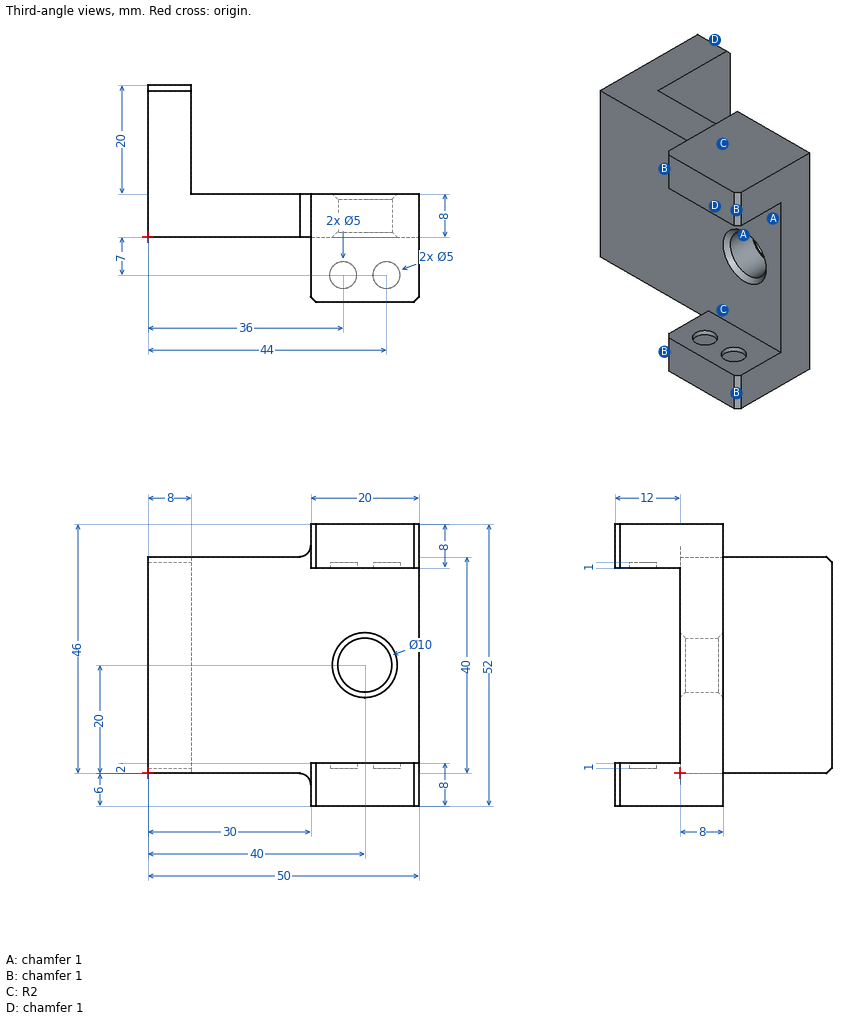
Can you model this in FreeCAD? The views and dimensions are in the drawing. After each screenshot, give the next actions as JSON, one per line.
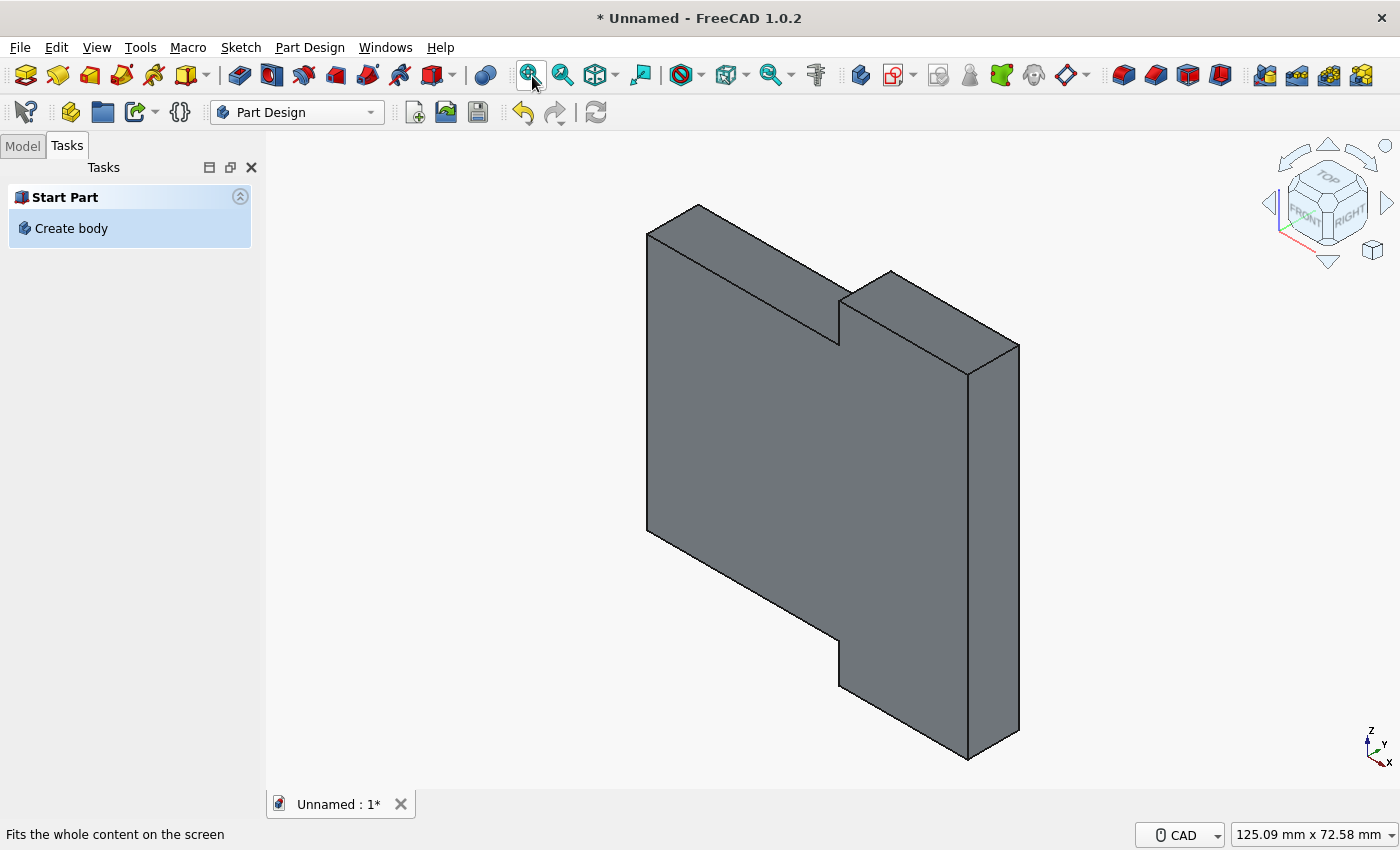
{"action": "left_click", "coordinate": [807, 474]}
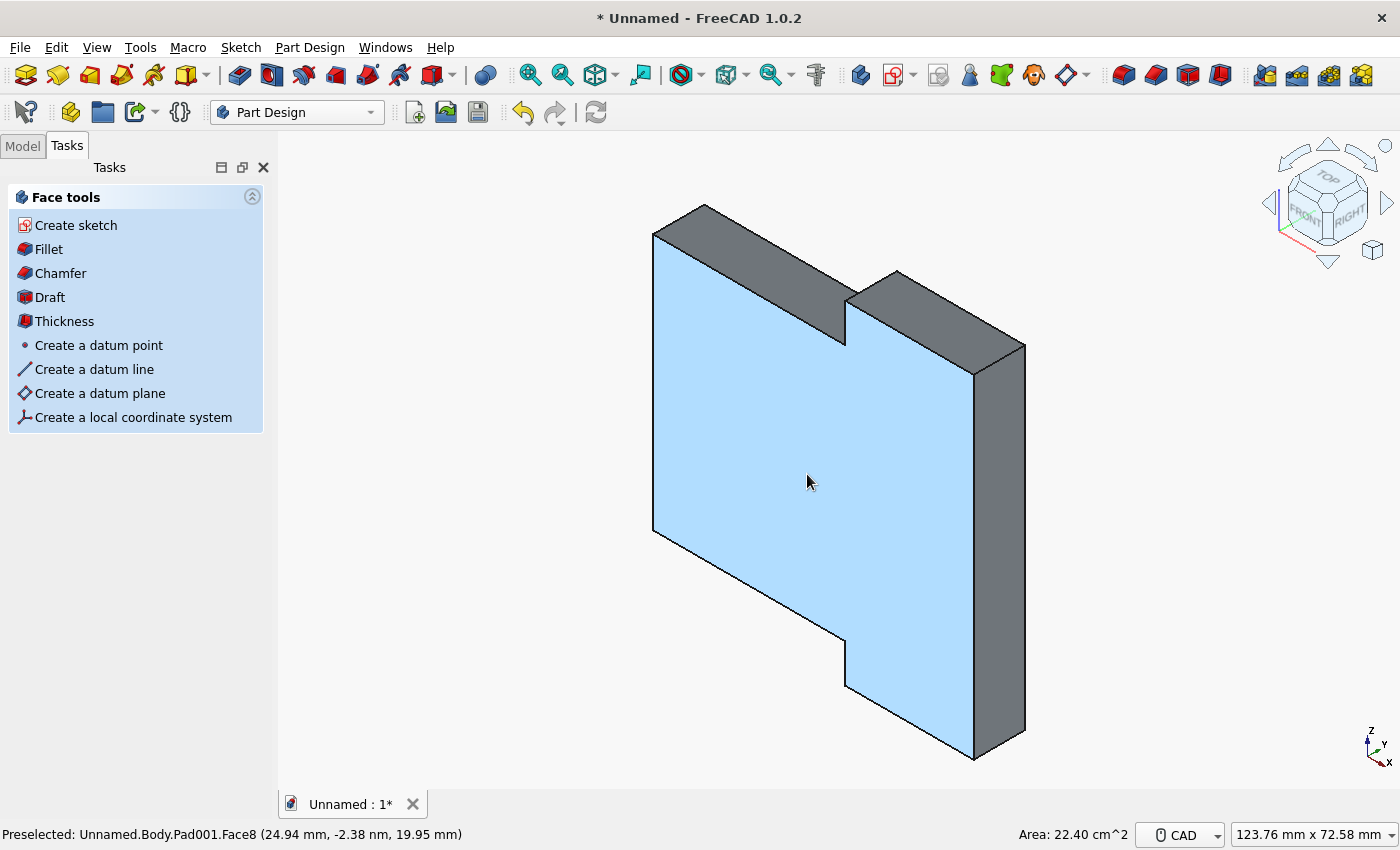
{"action": "left_click", "coordinate": [894, 76]}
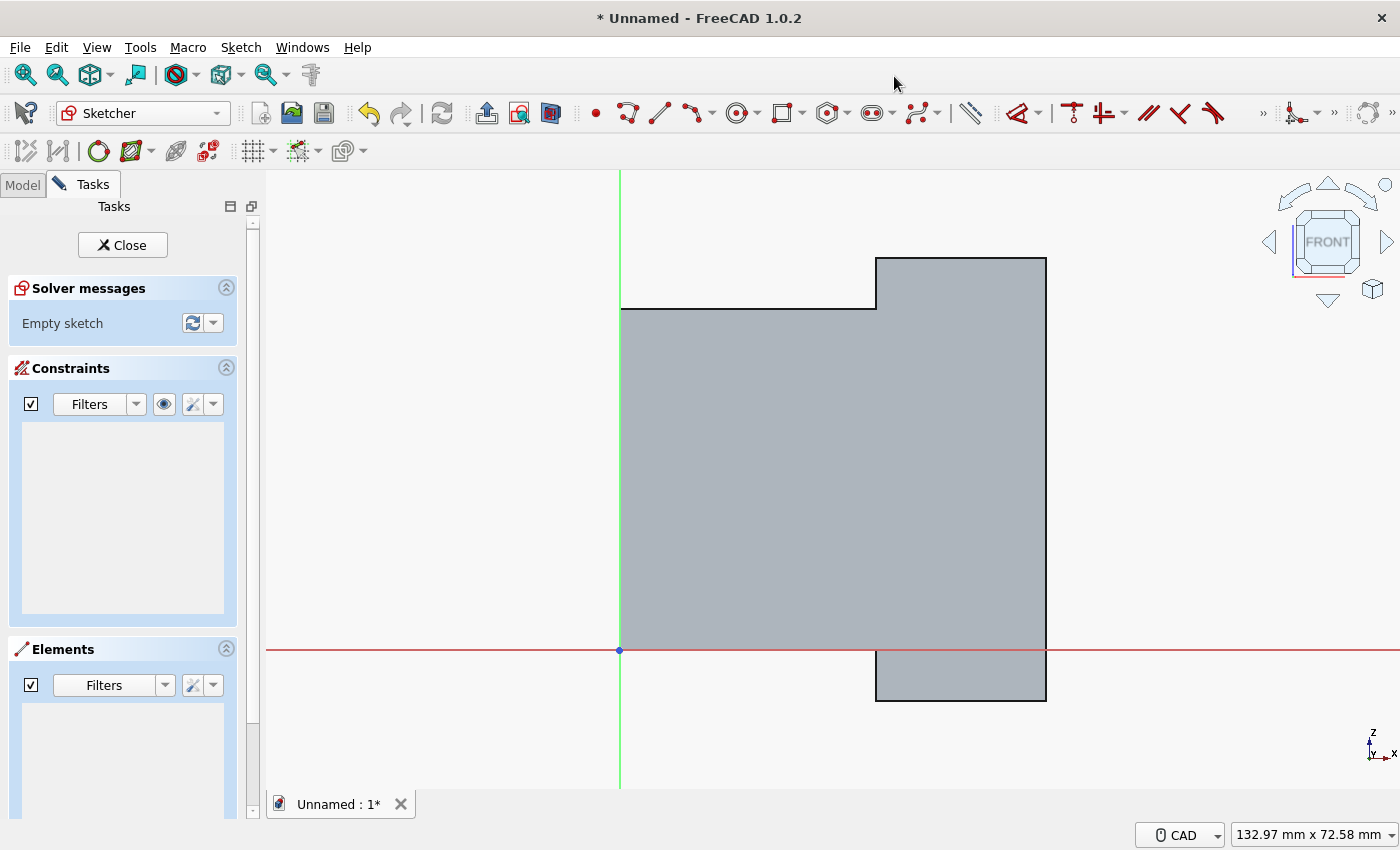
{"action": "scroll", "coordinate": [1011, 480], "scroll_direction": "up", "scroll_amount": 8}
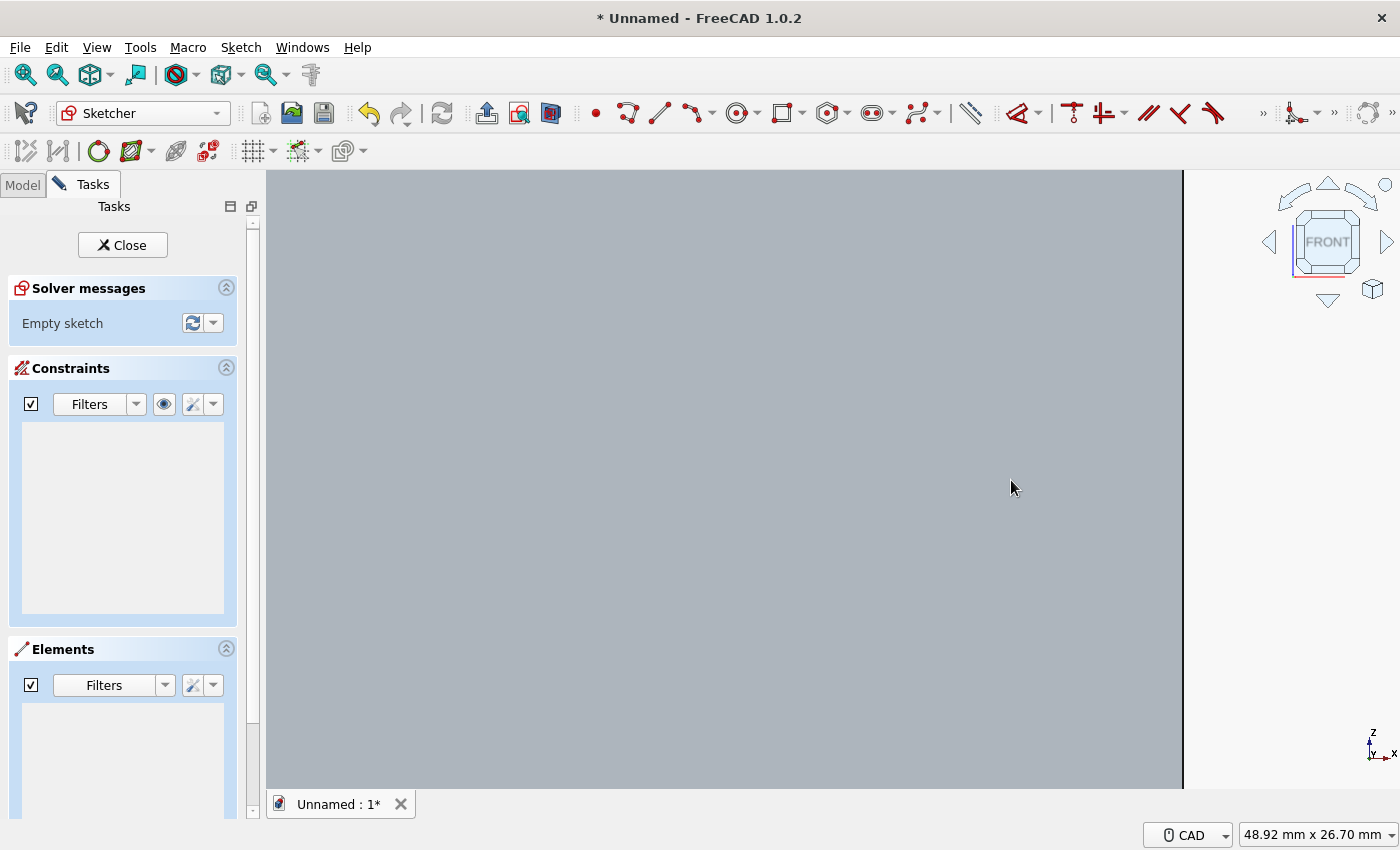
{"action": "left_click", "coordinate": [738, 114]}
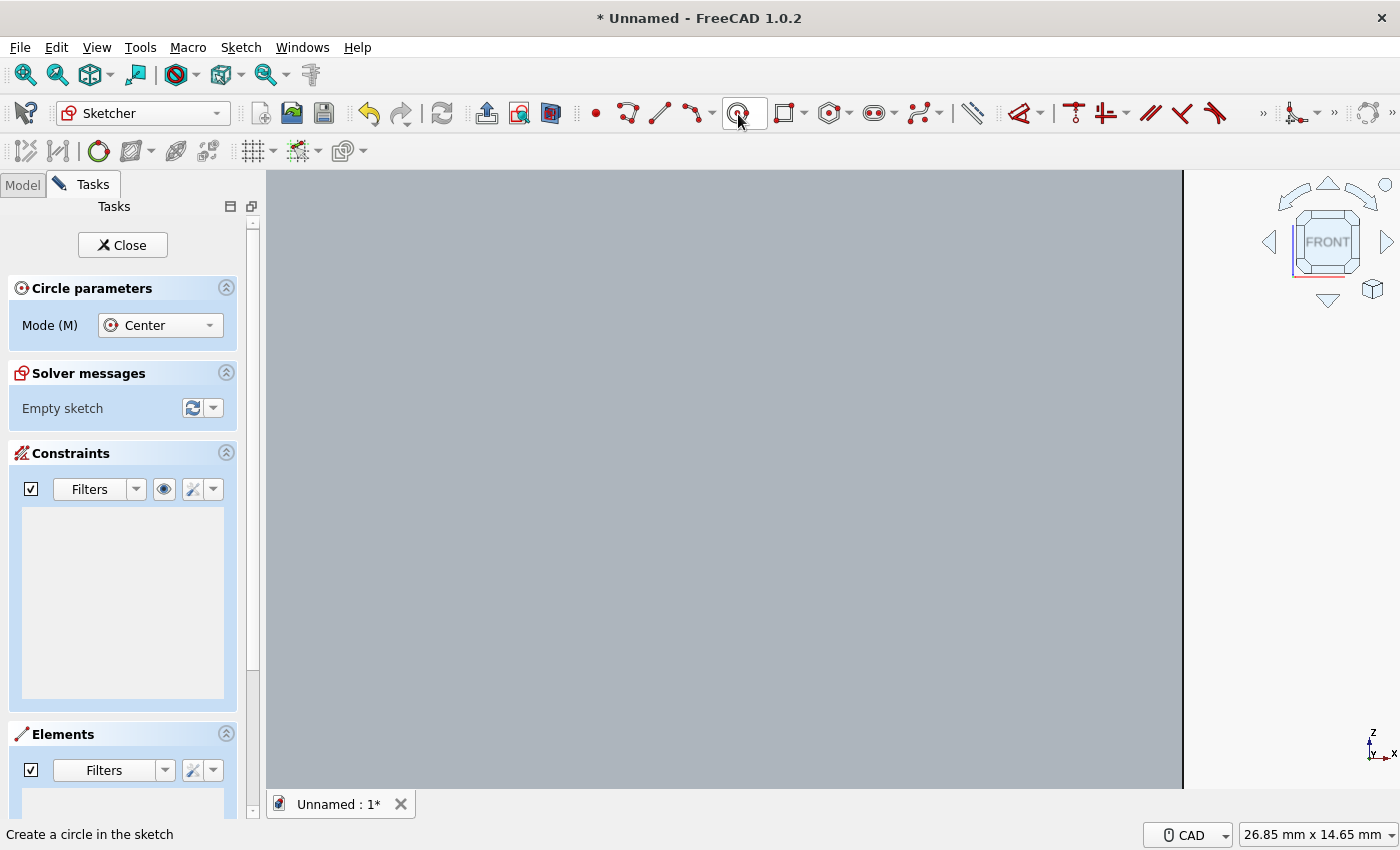
{"action": "left_click", "coordinate": [760, 476]}
{"action": "mouse_move", "coordinate": [910, 326]}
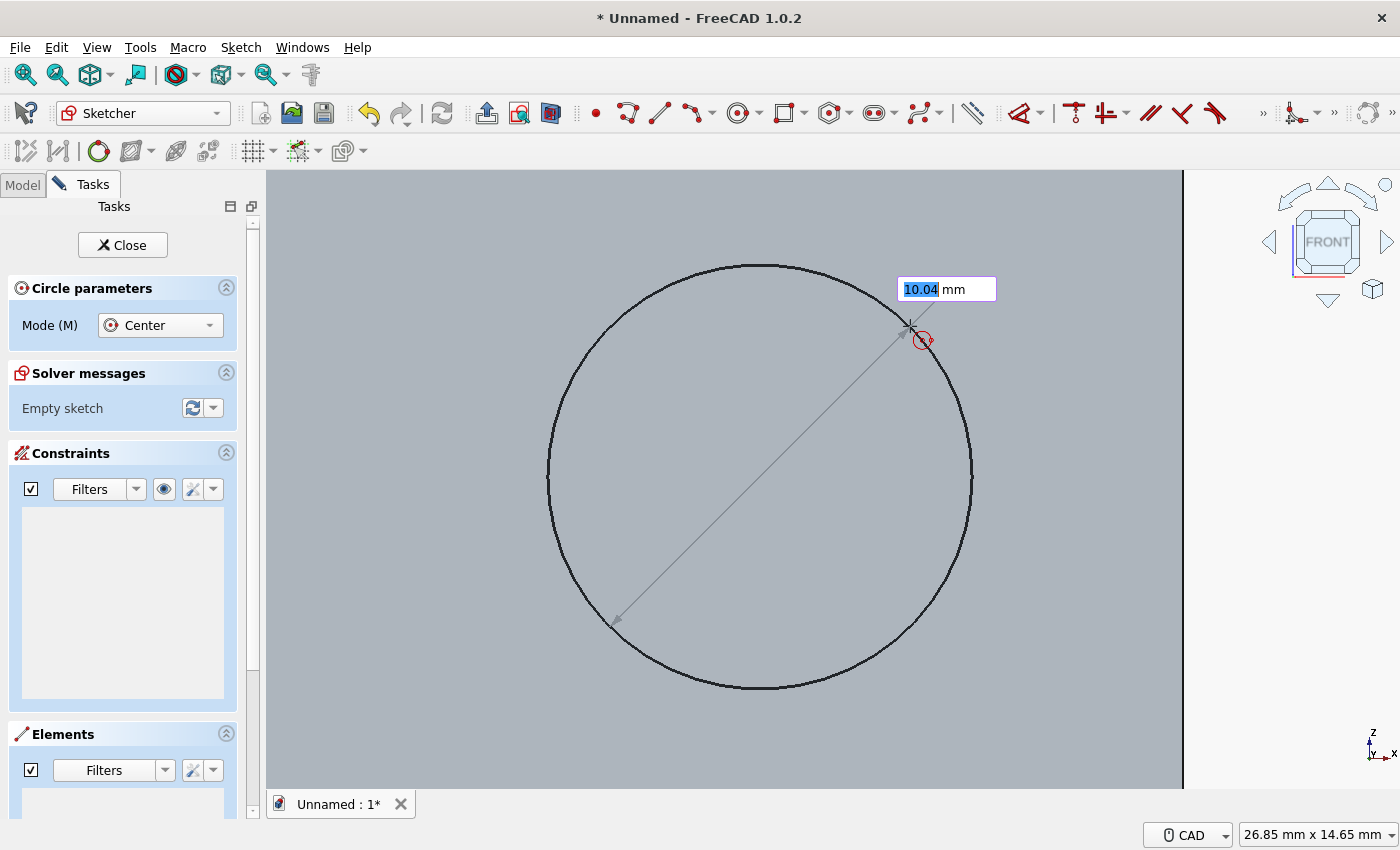
{"action": "type", "text": "10"}
{"action": "key", "text": "Return"}
{"action": "key", "text": "Escape"}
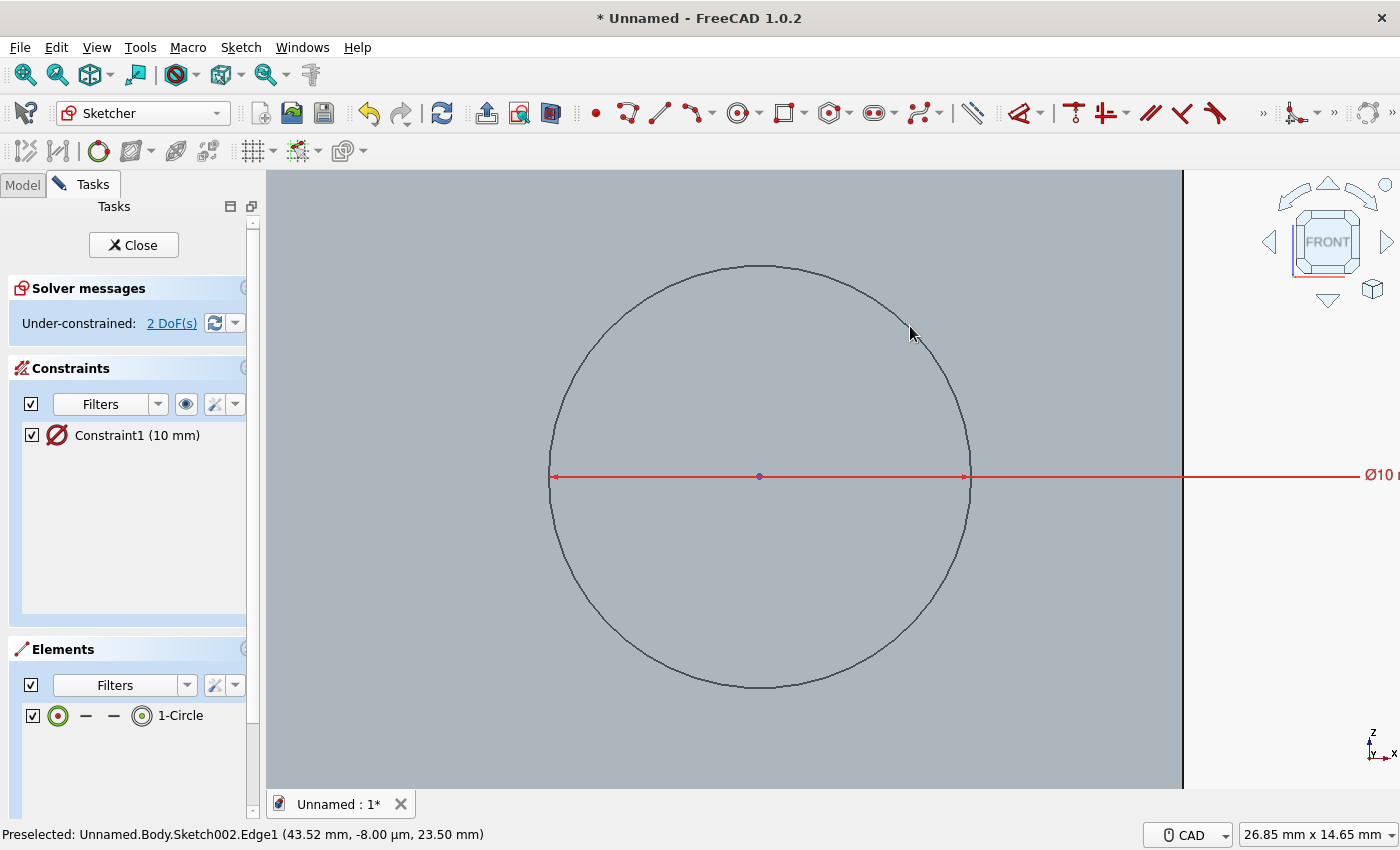
{"action": "left_click", "coordinate": [1020, 114]}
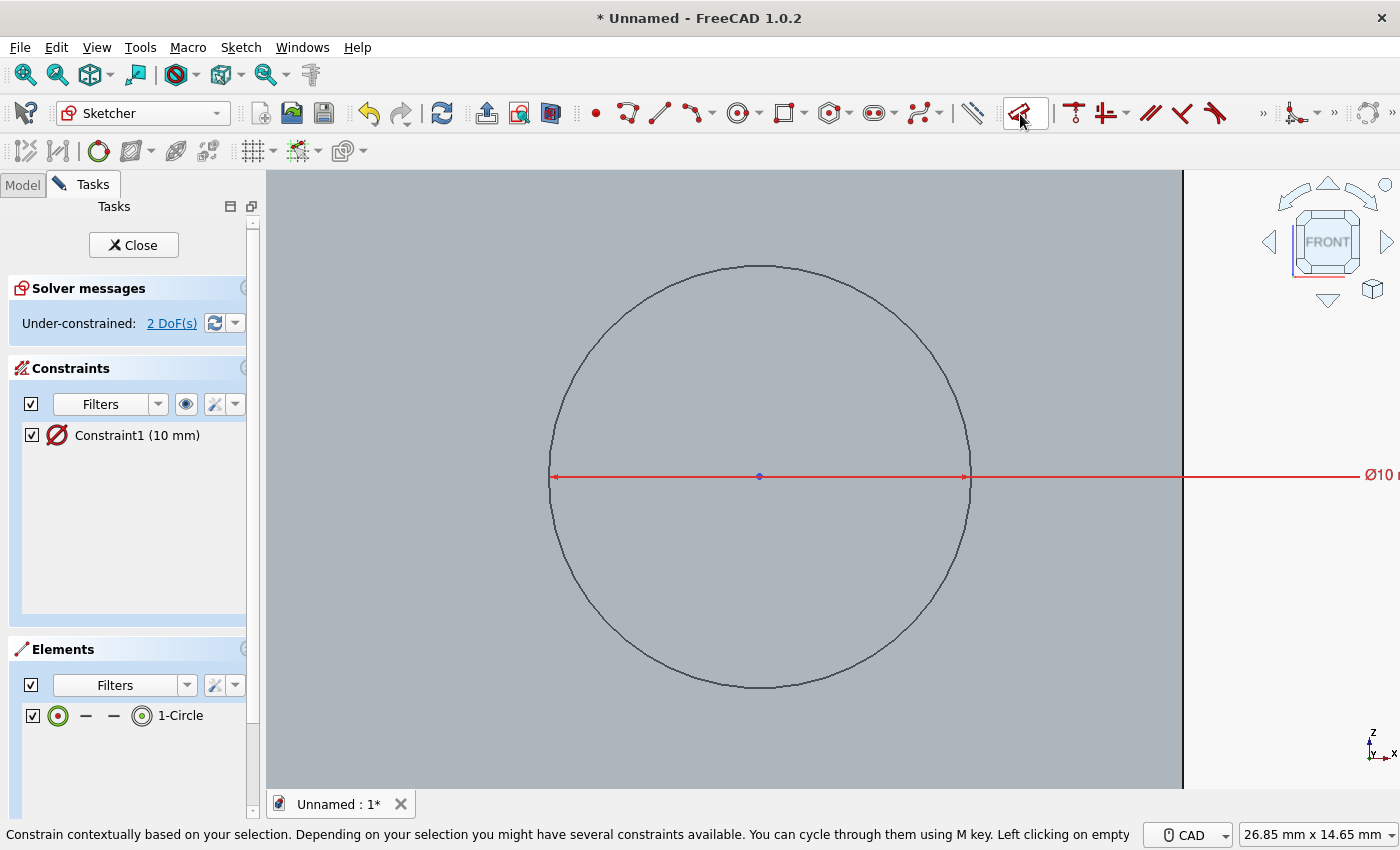
{"action": "left_click", "coordinate": [760, 477]}
{"action": "left_click", "coordinate": [527, 443]}